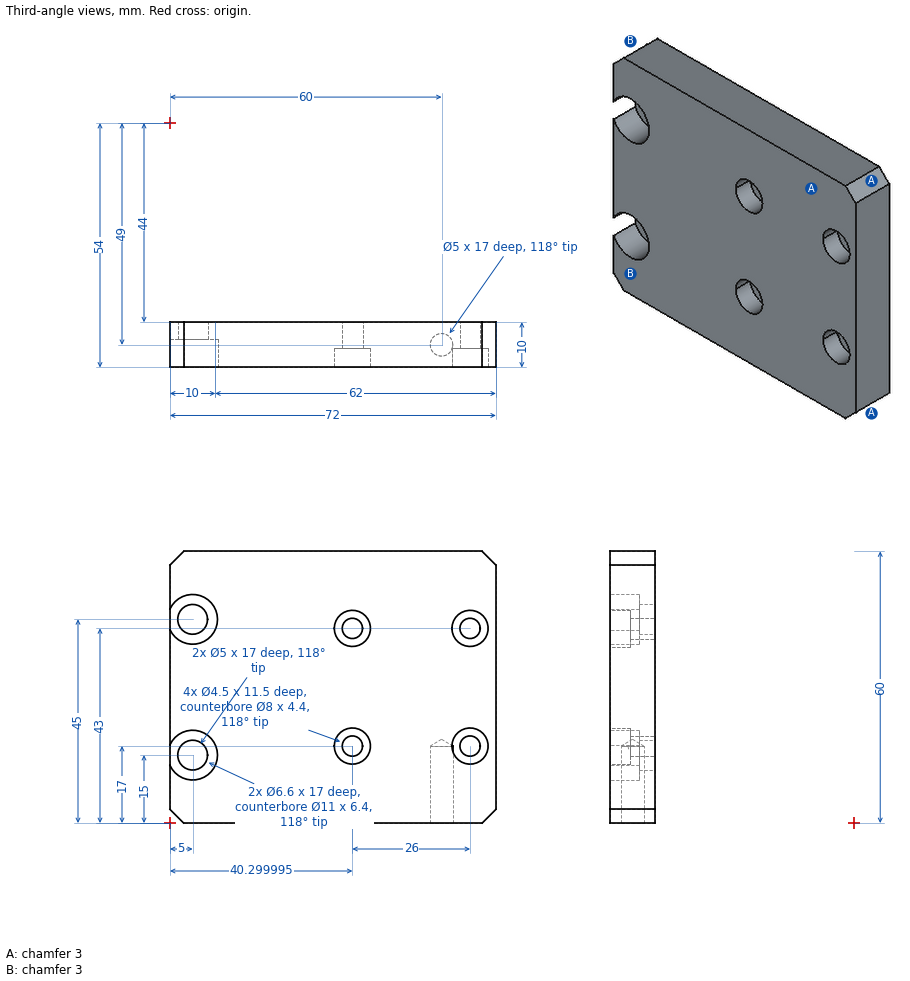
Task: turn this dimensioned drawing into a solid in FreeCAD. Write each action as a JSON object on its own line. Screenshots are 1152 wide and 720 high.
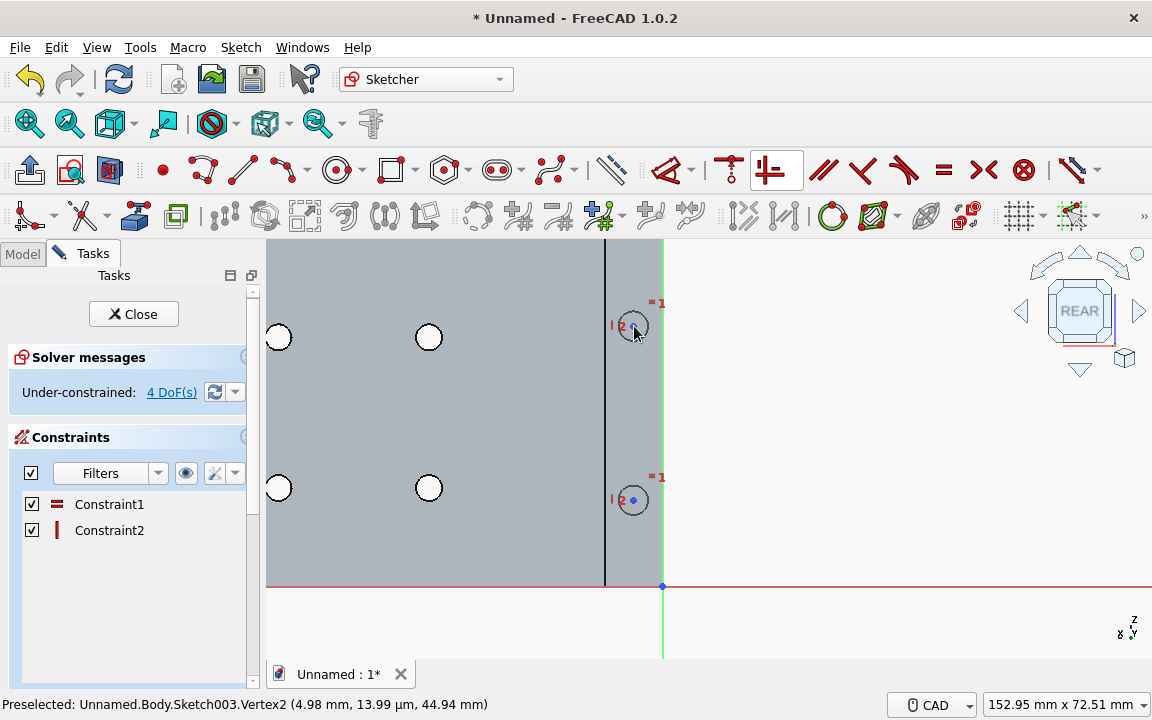
{"action": "left_click", "coordinate": [666, 170]}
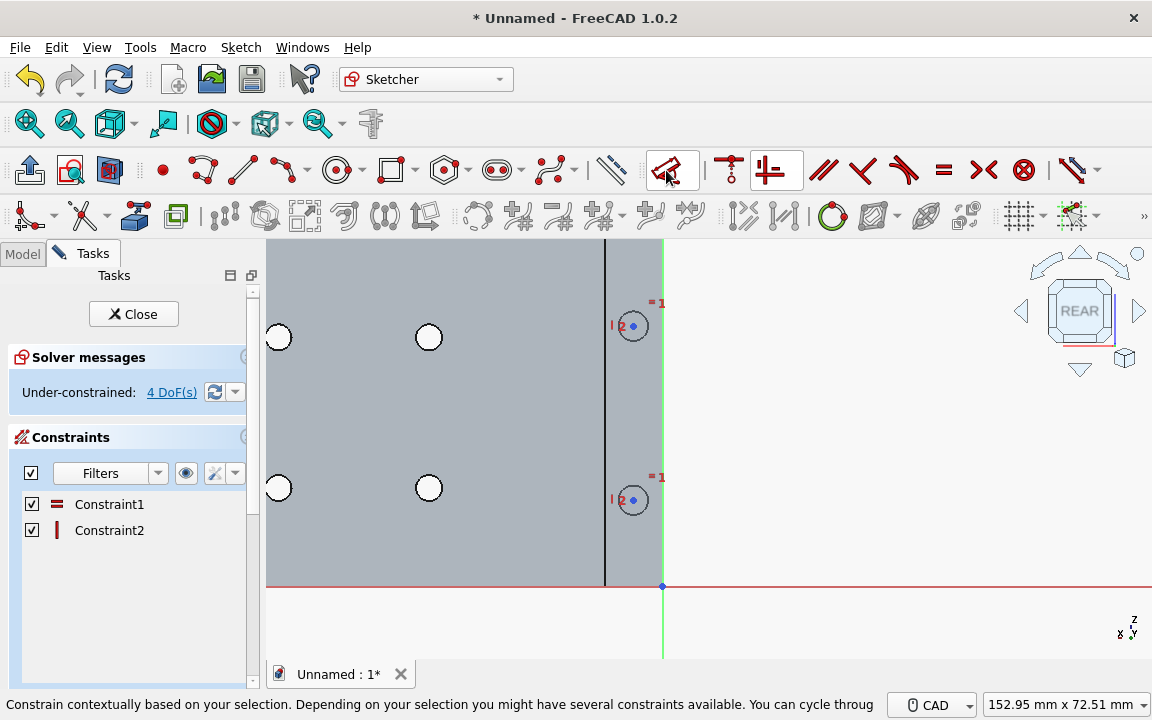
{"action": "scroll", "coordinate": [644, 490], "scroll_direction": "up", "scroll_amount": 2}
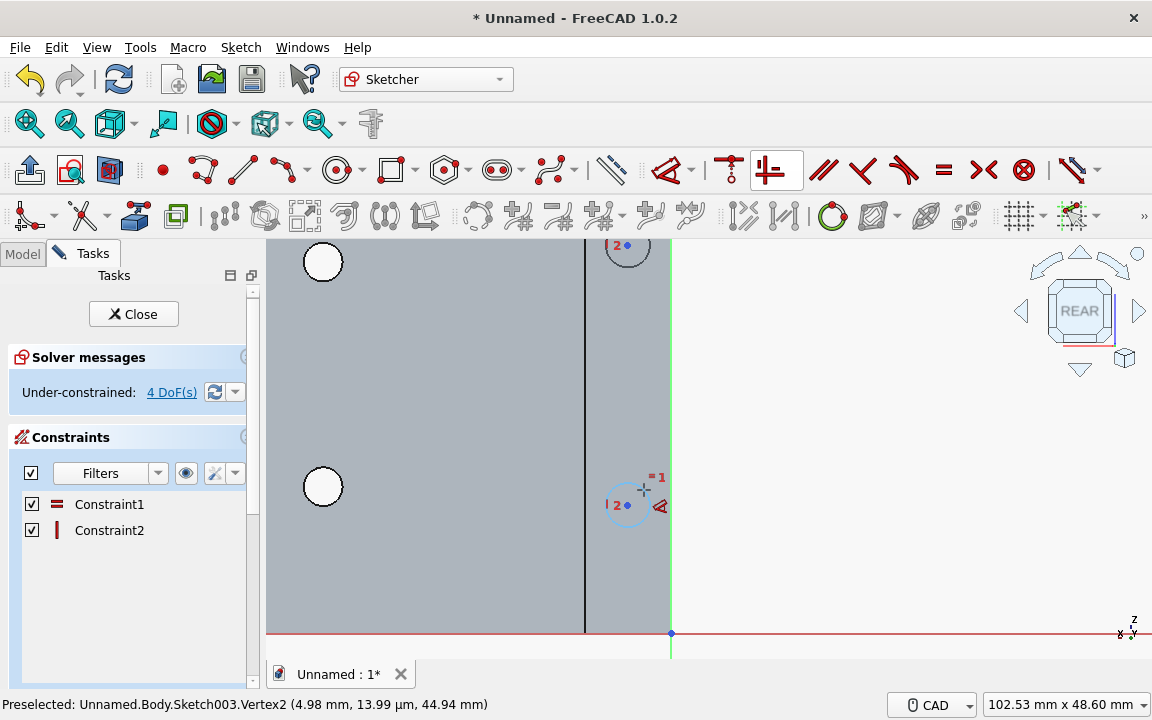
{"action": "left_click", "coordinate": [643, 489]}
{"action": "left_click", "coordinate": [642, 453]}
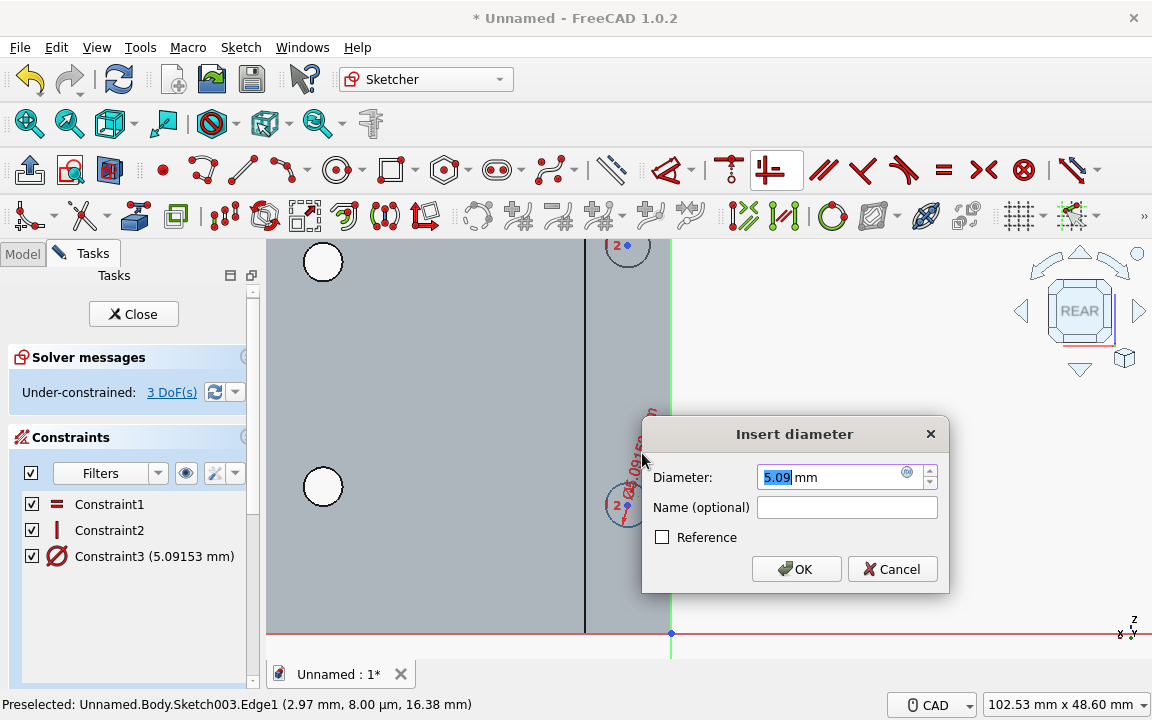
{"action": "type", "text": "5"}
{"action": "key", "text": "Return"}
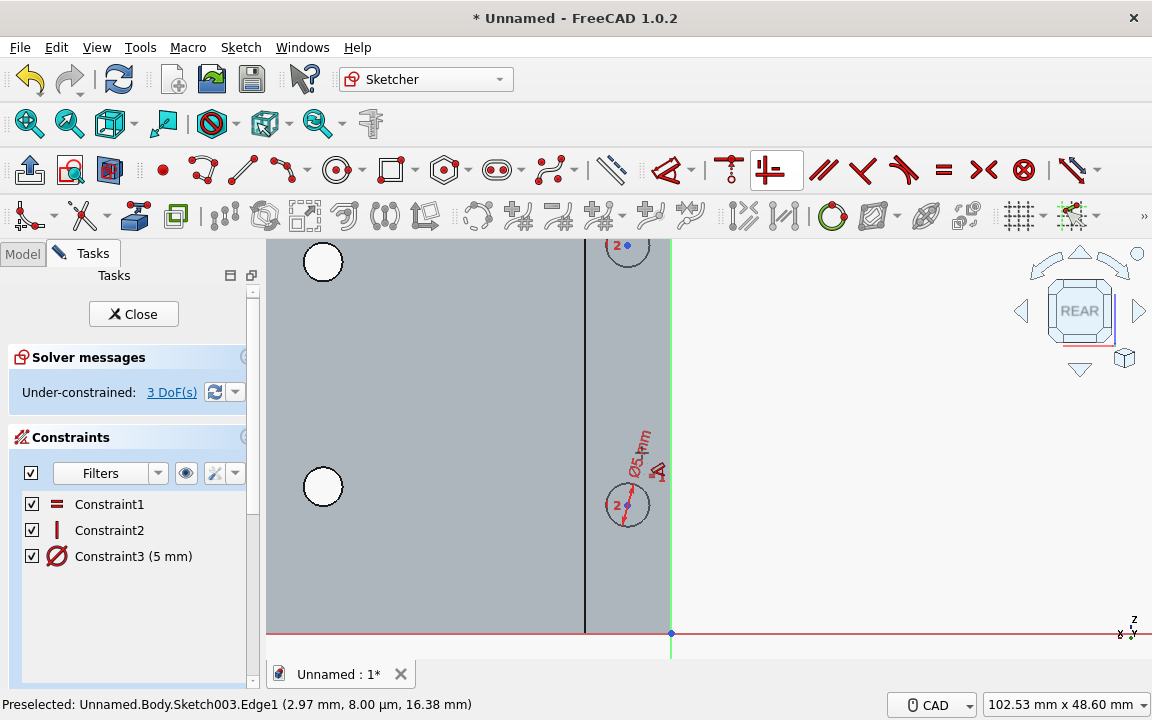
{"action": "left_click", "coordinate": [628, 505]}
{"action": "left_click", "coordinate": [650, 423]}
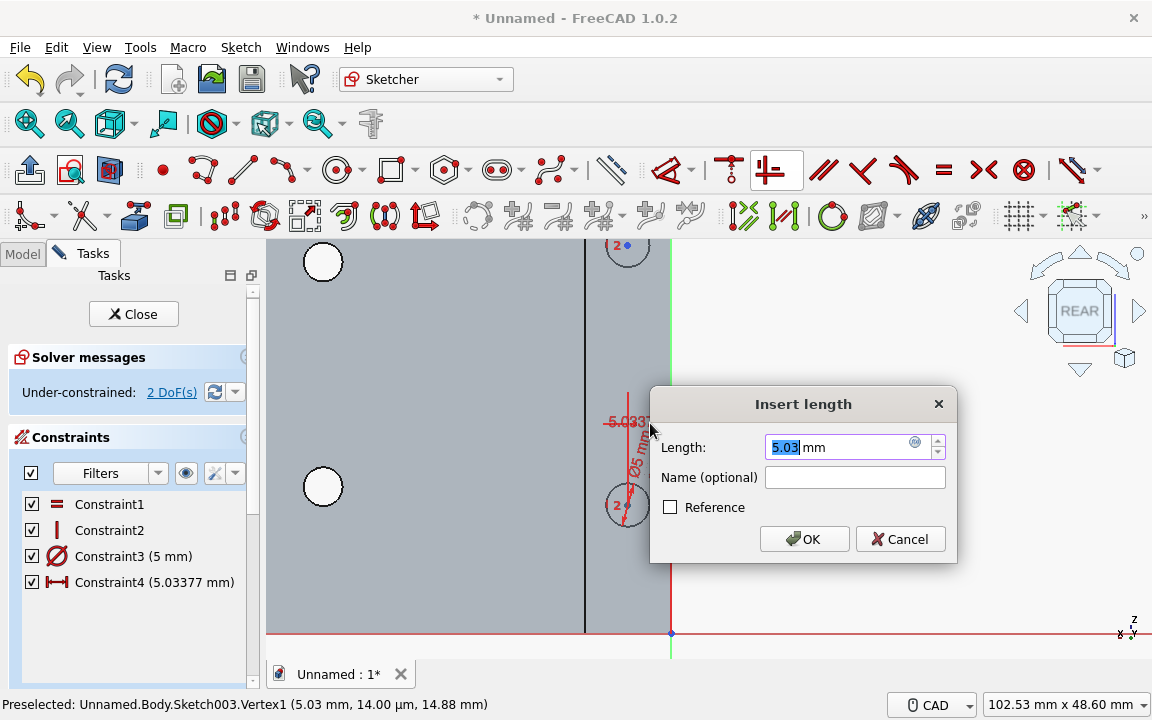
{"action": "type", "text": "5"}
{"action": "key", "text": "Return"}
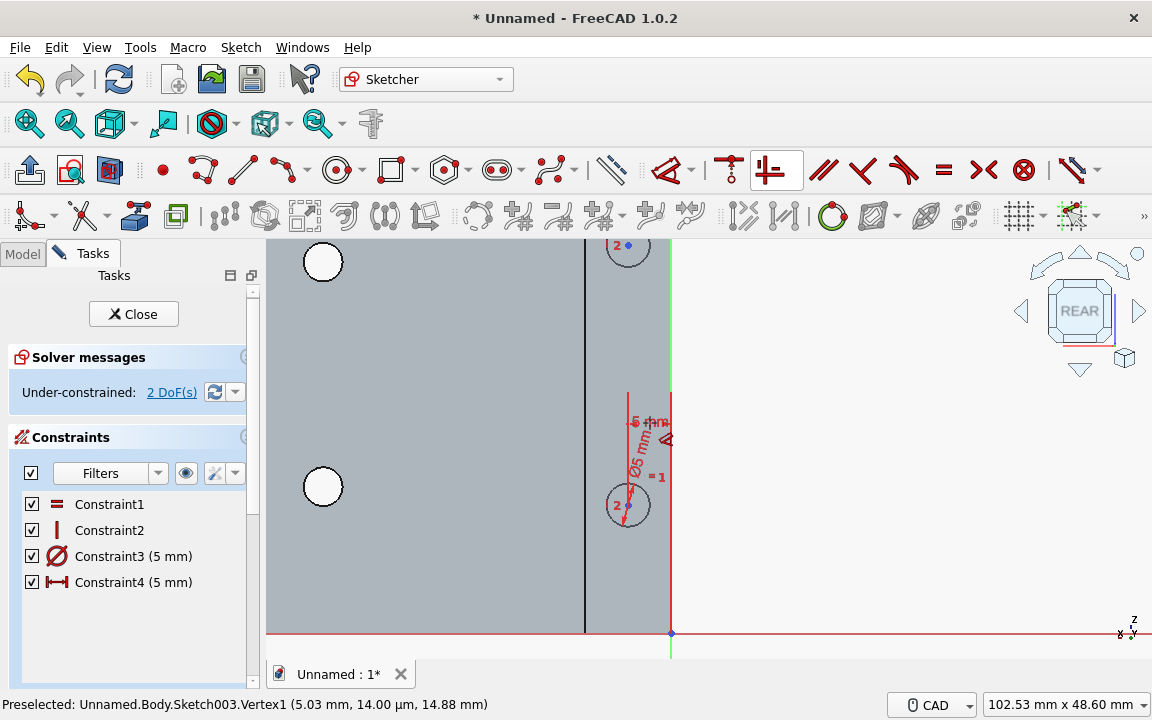
{"action": "left_click", "coordinate": [628, 505]}
{"action": "left_click", "coordinate": [705, 568]}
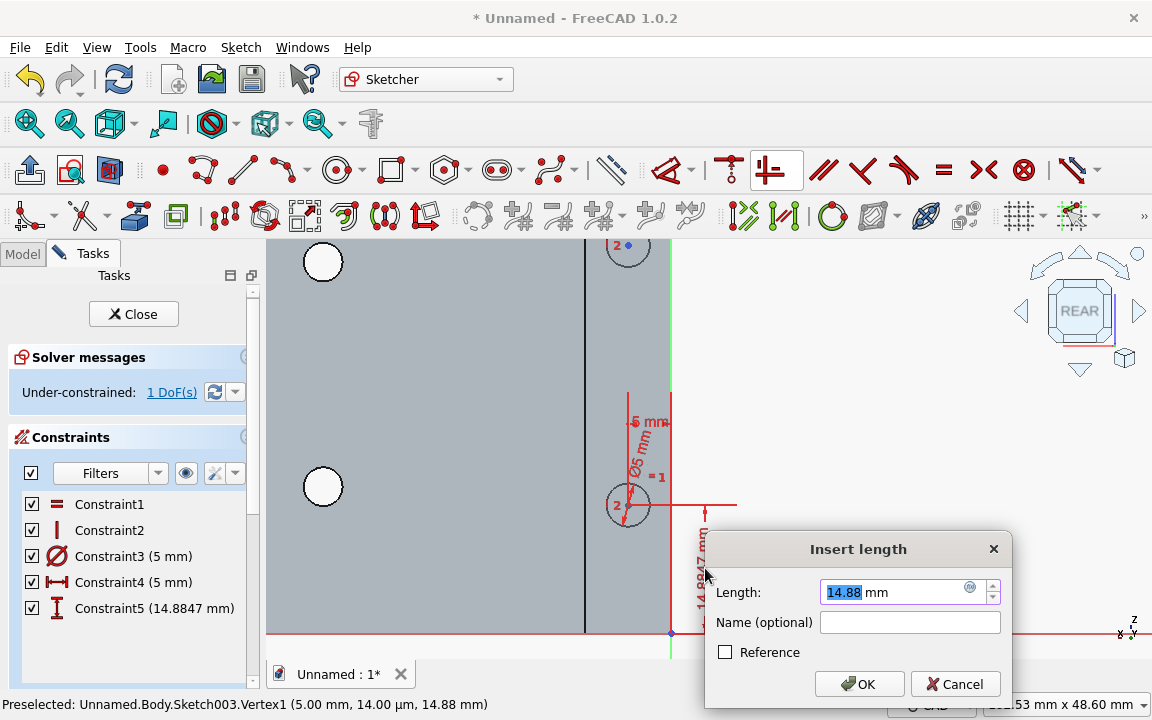
{"action": "type", "text": "15"}
{"action": "key", "text": "Return"}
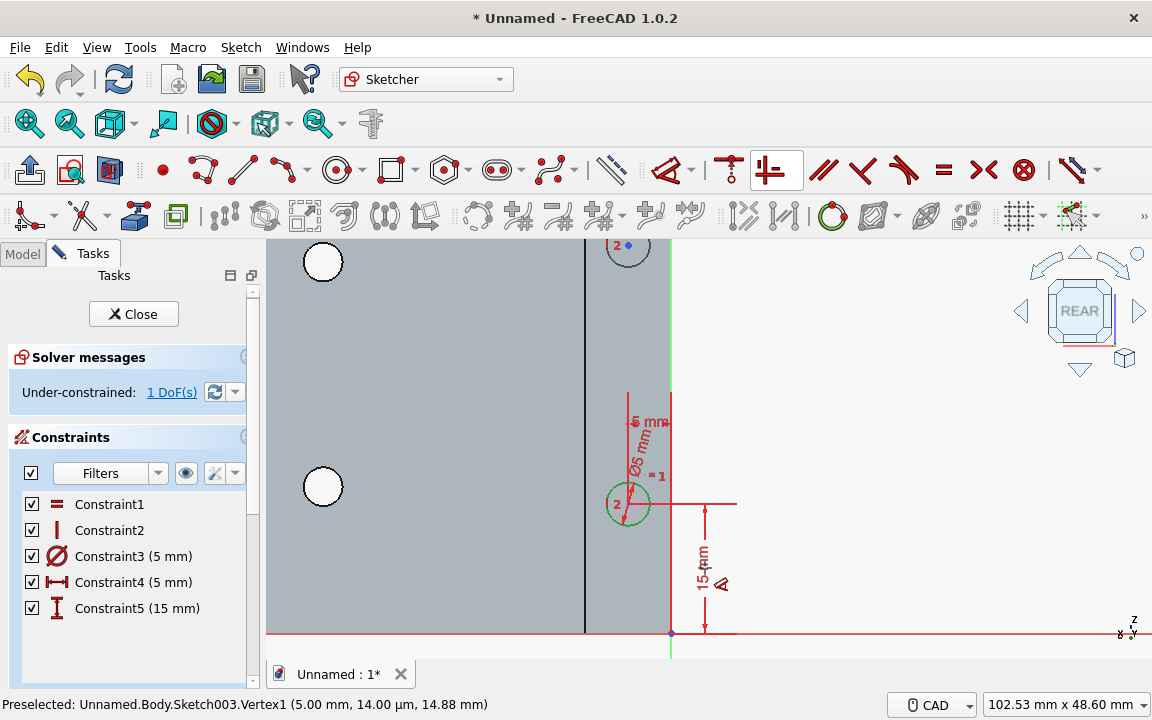
{"action": "scroll", "coordinate": [644, 491], "scroll_direction": "down", "scroll_amount": 2}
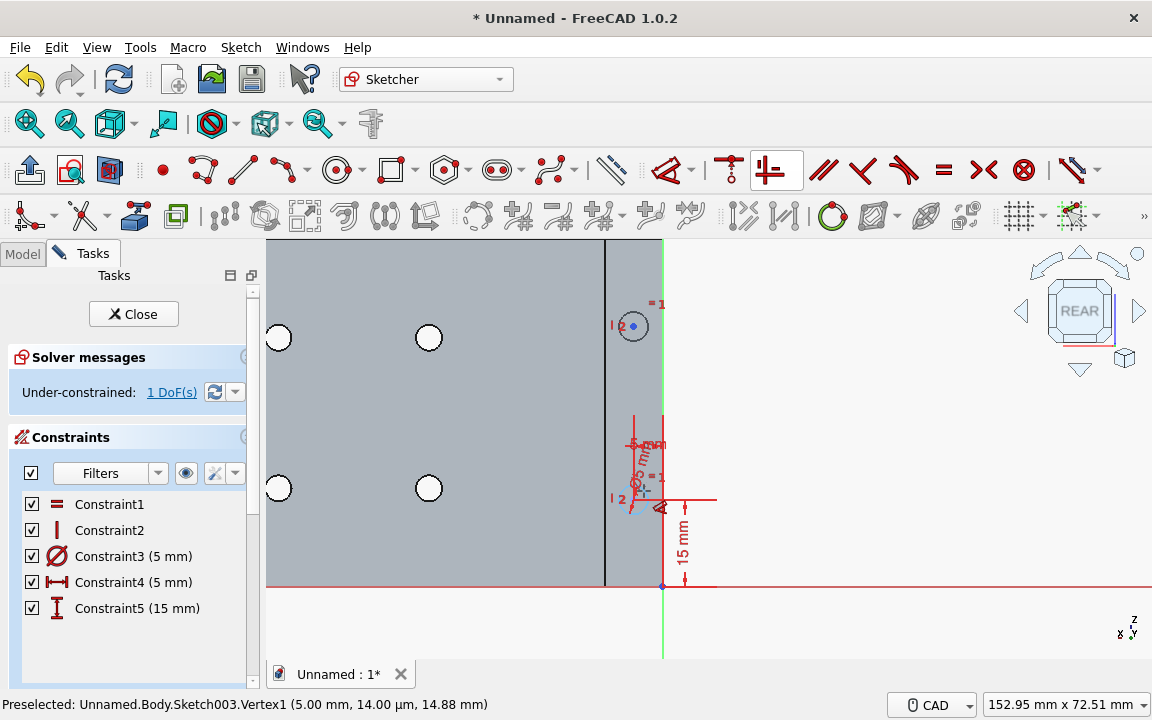
{"action": "left_click", "coordinate": [634, 327]}
{"action": "left_click", "coordinate": [697, 397]}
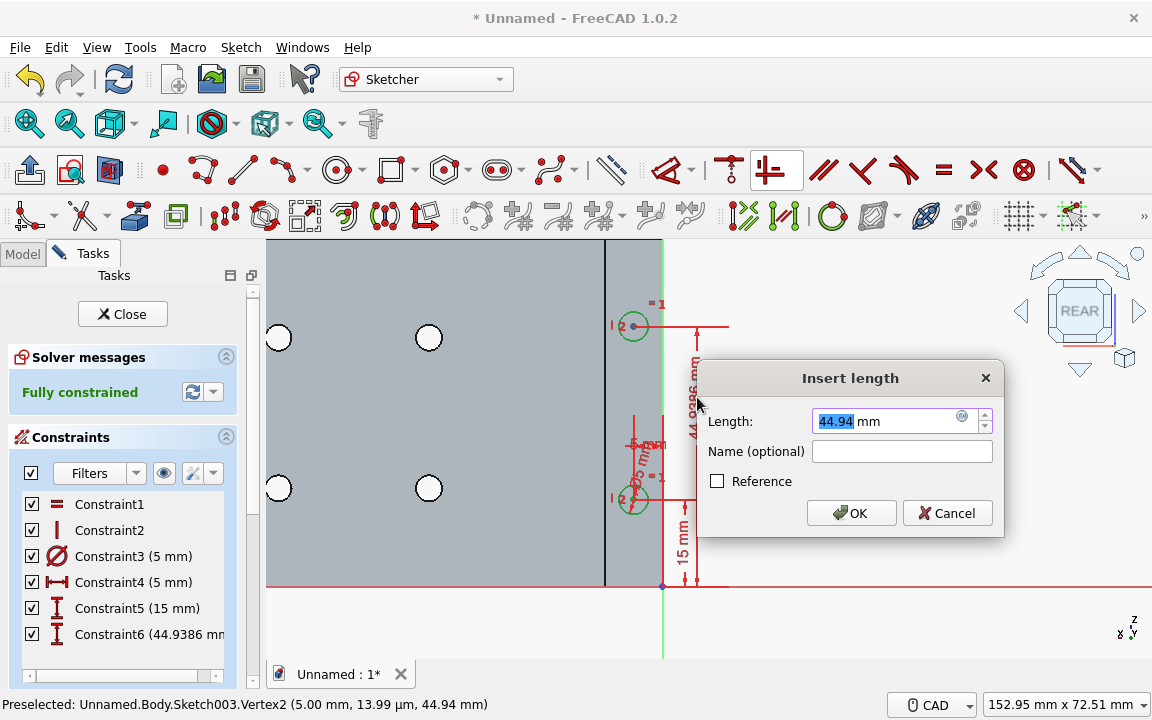
{"action": "type", "text": "45"}
{"action": "key", "text": "Return"}
{"action": "key", "text": "Escape"}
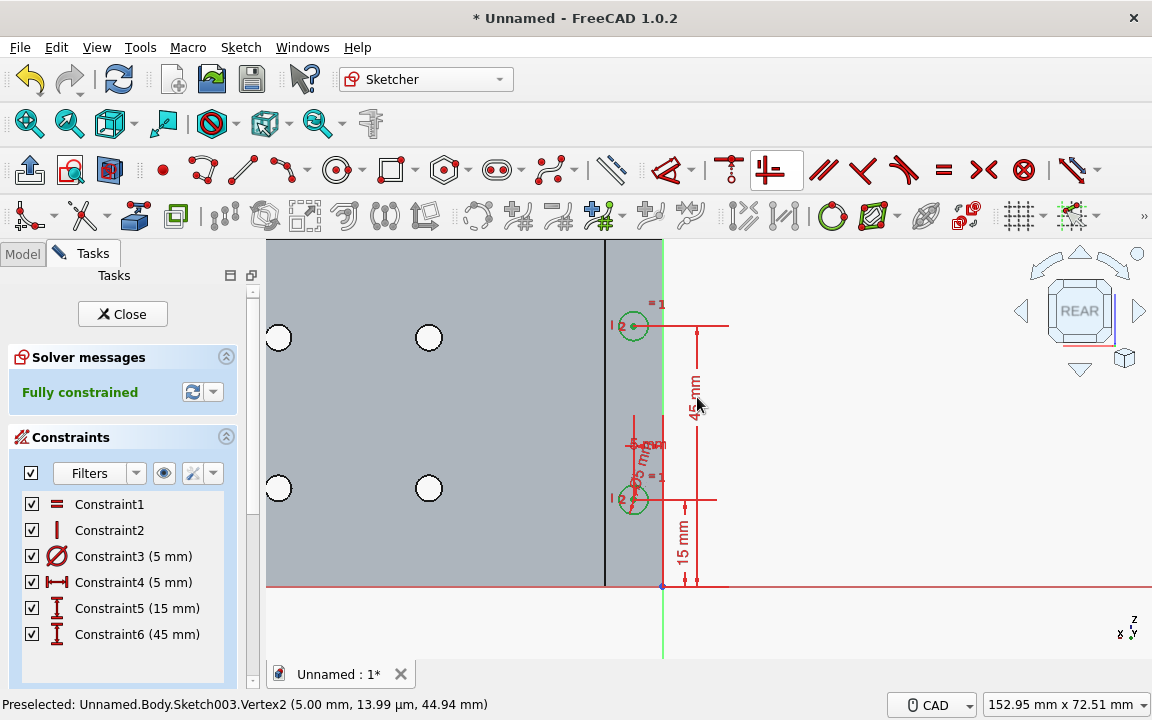
{"action": "left_click", "coordinate": [123, 314]}